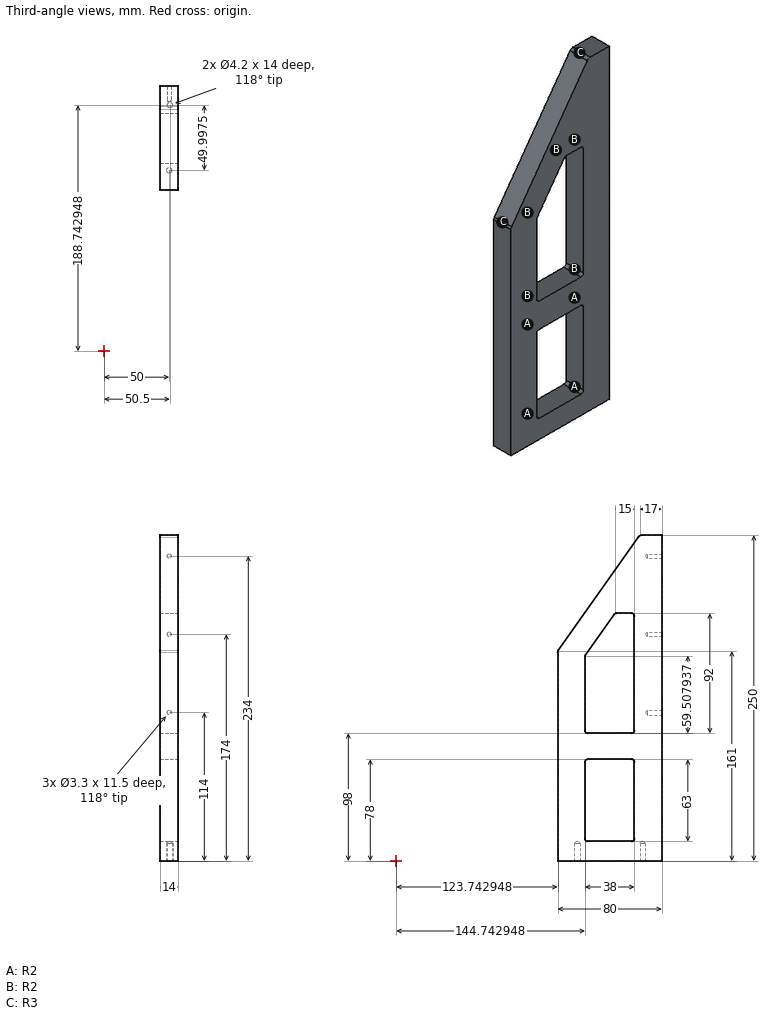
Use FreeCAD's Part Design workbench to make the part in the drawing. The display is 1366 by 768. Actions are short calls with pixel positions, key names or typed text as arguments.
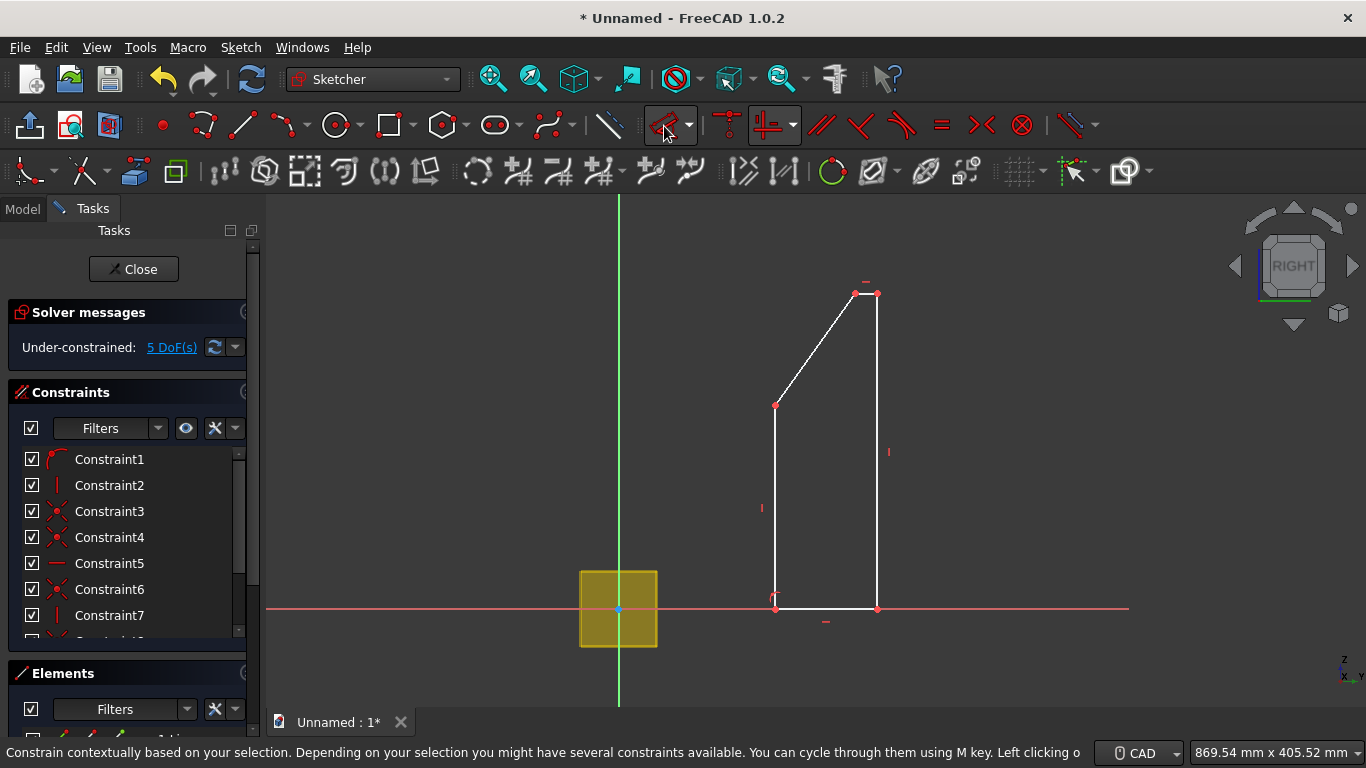
scroll(866, 294, up, 4)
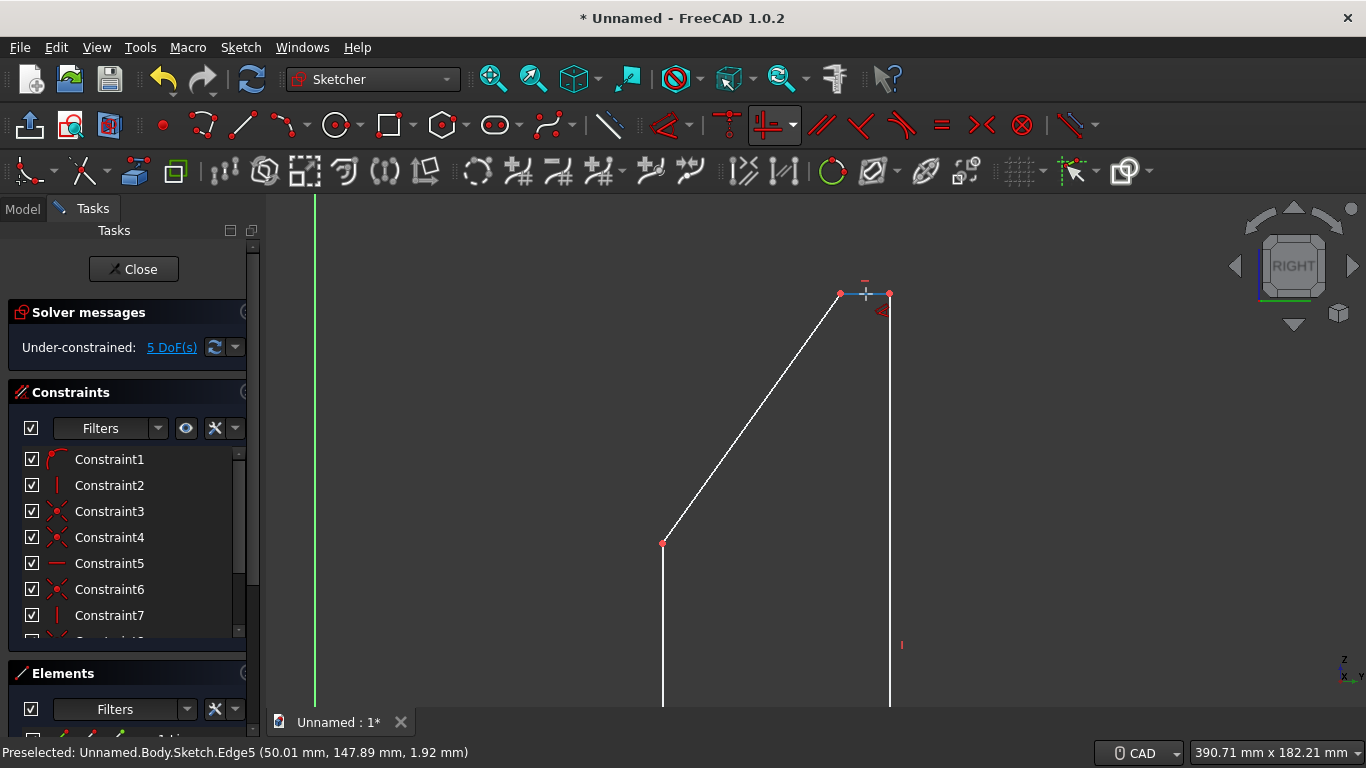
click(865, 294)
click(865, 260)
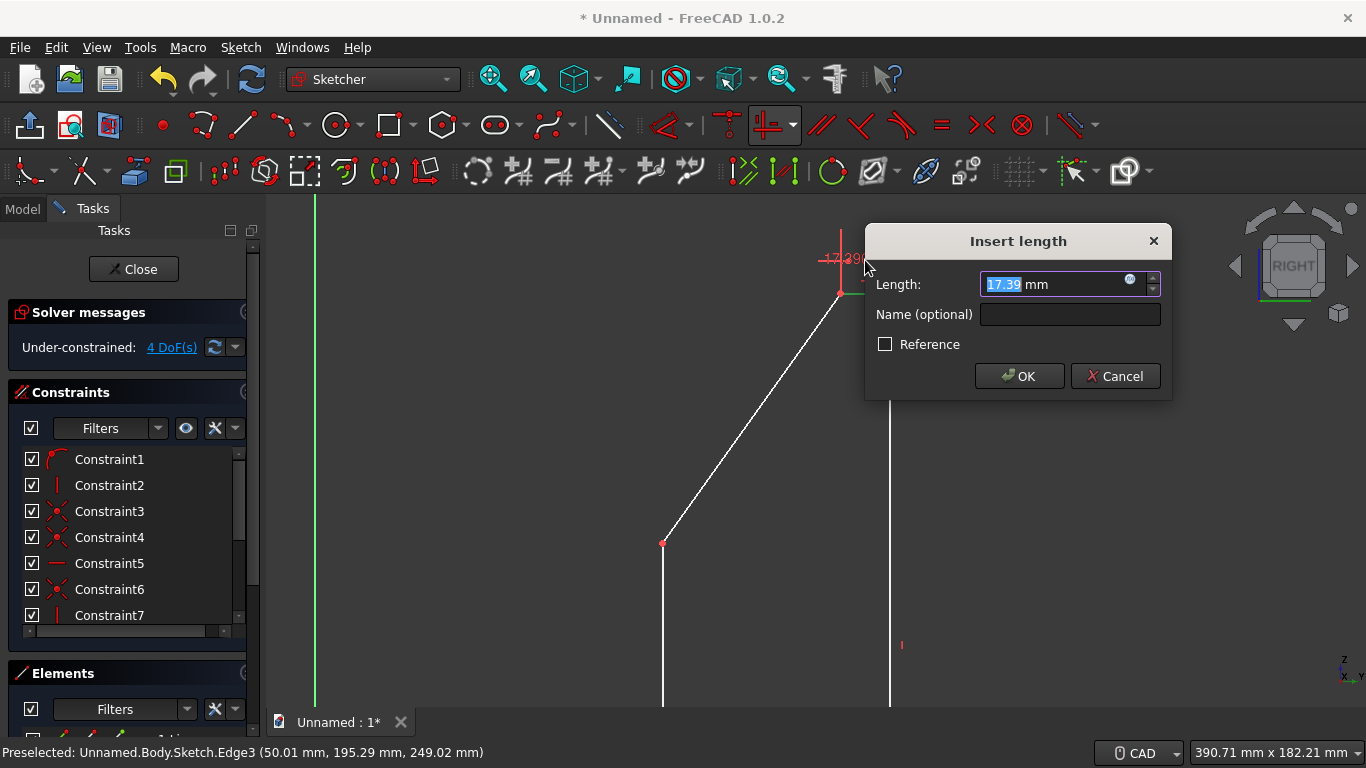
text(17)
key(Return)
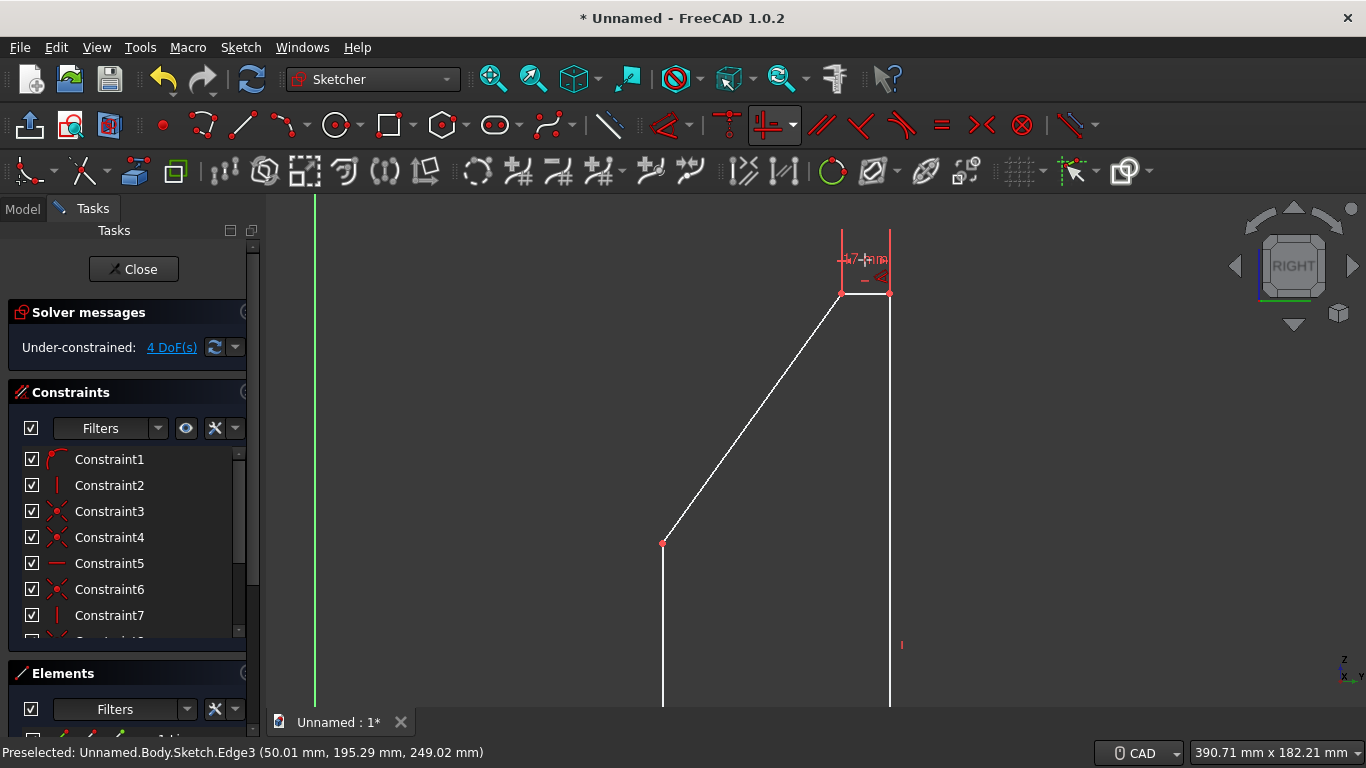
scroll(866, 293, down, 4)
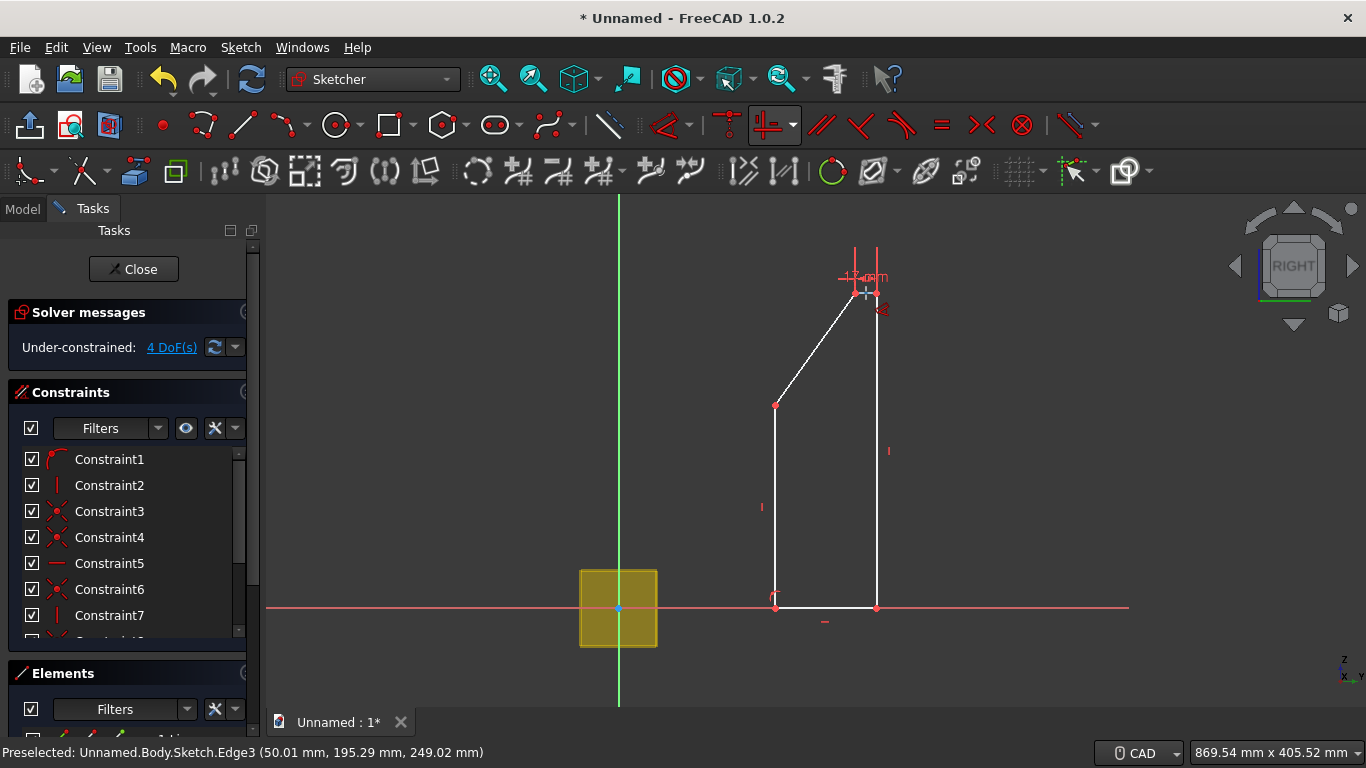
click(846, 608)
click(826, 642)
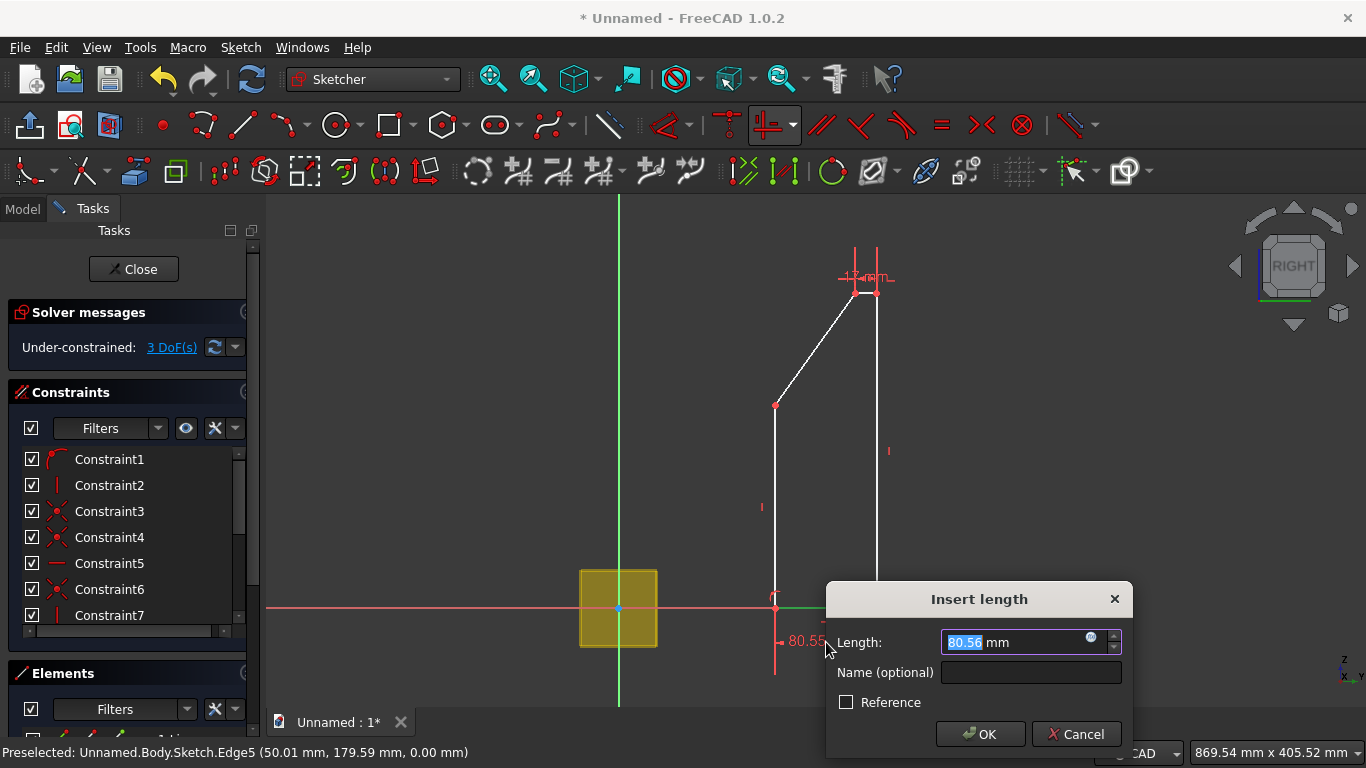
text(80)
key(Return)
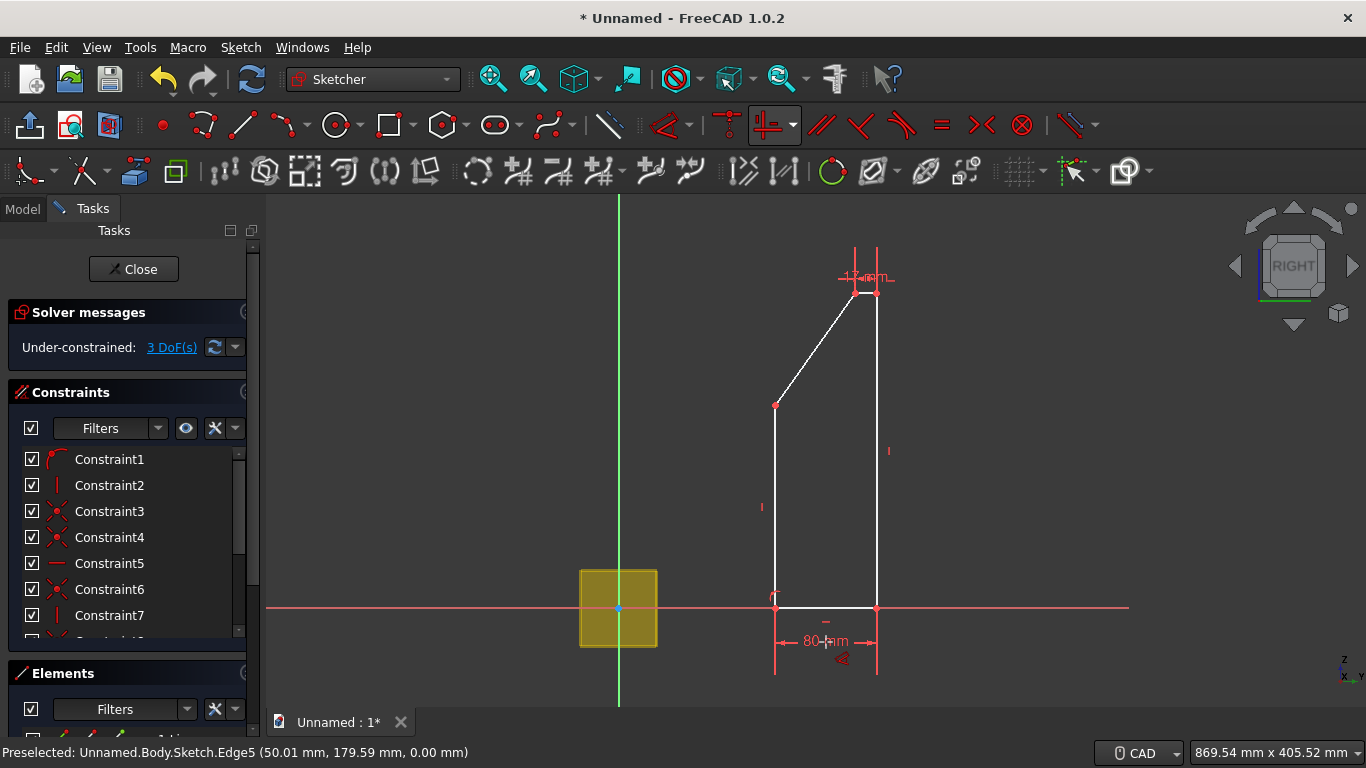
click(775, 548)
click(809, 507)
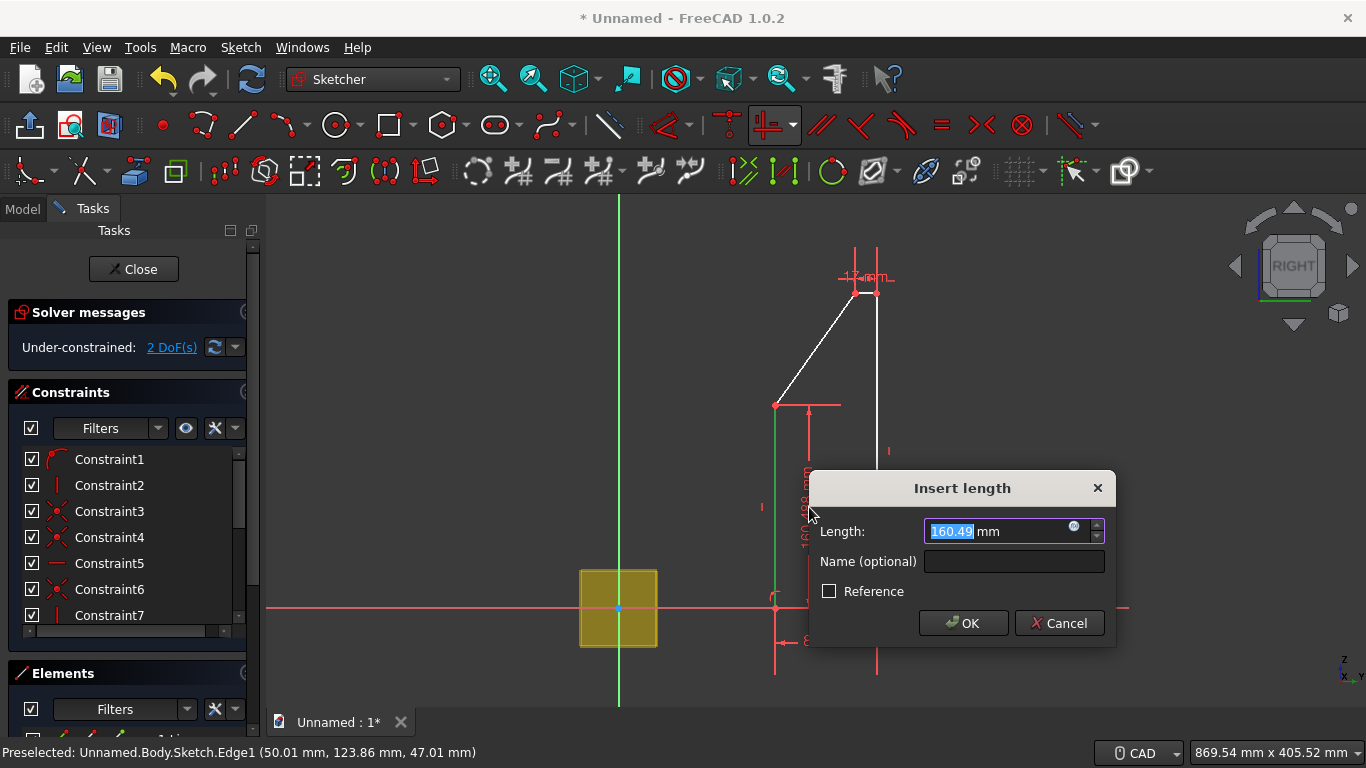
text(161)
key(Return)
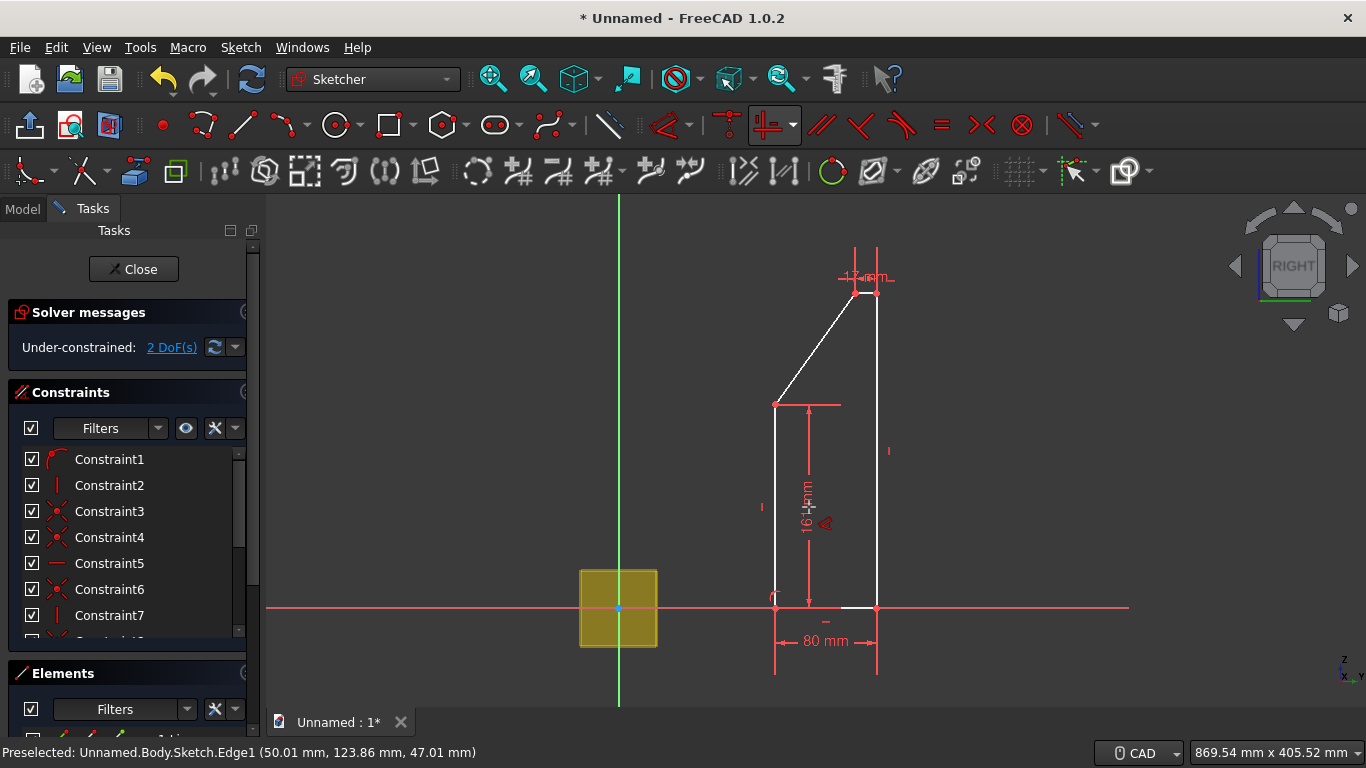
click(877, 388)
click(911, 451)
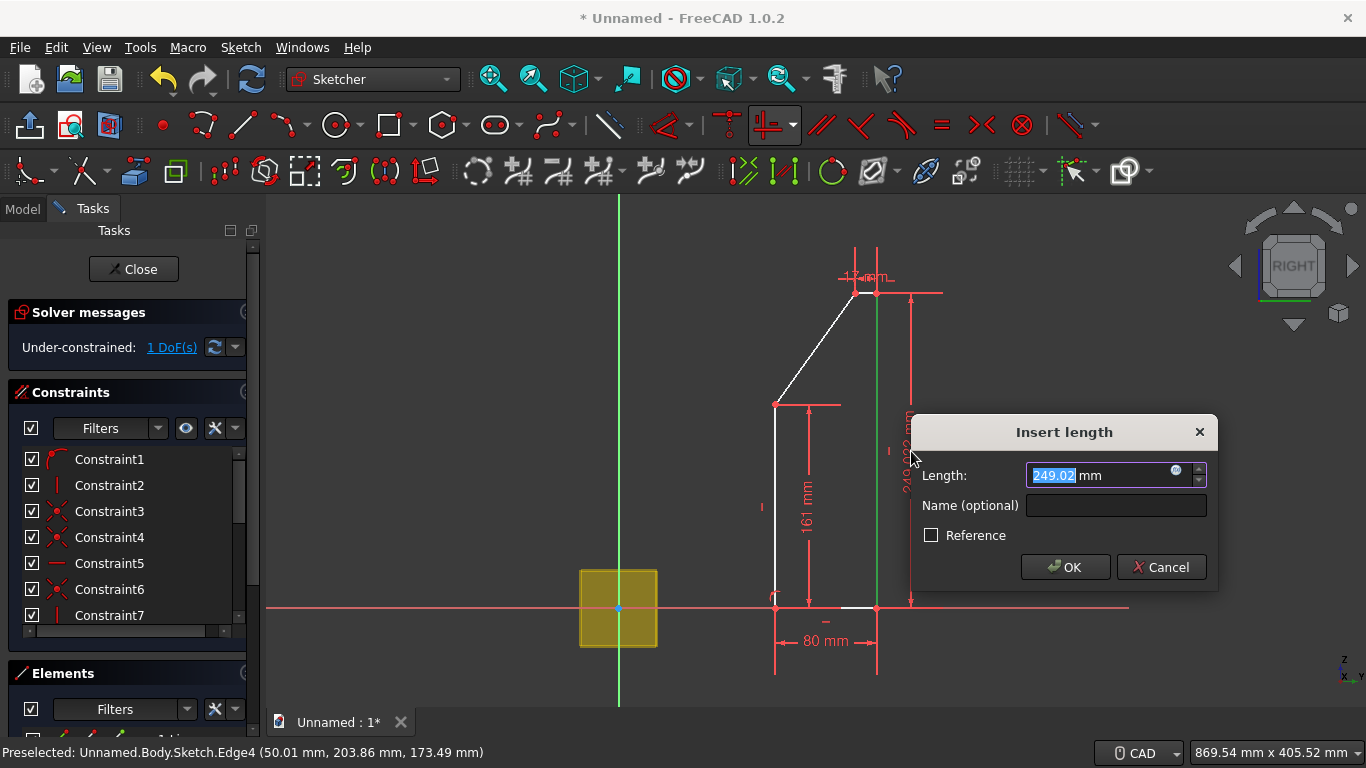
text(250)
key(Return)